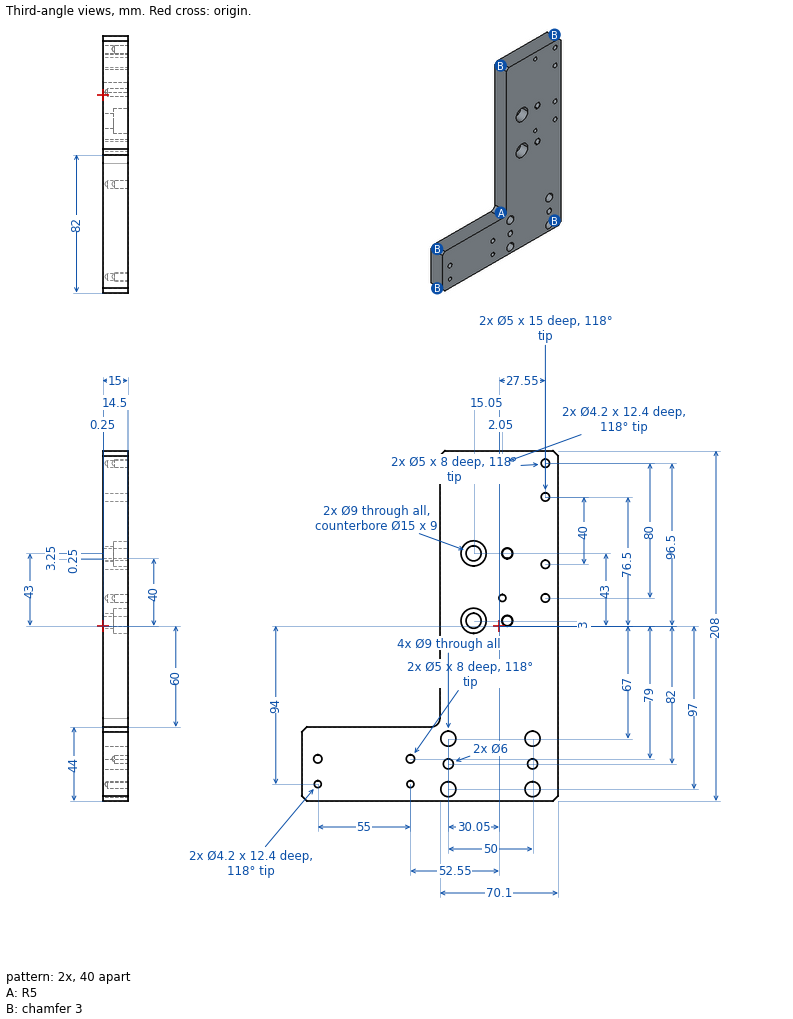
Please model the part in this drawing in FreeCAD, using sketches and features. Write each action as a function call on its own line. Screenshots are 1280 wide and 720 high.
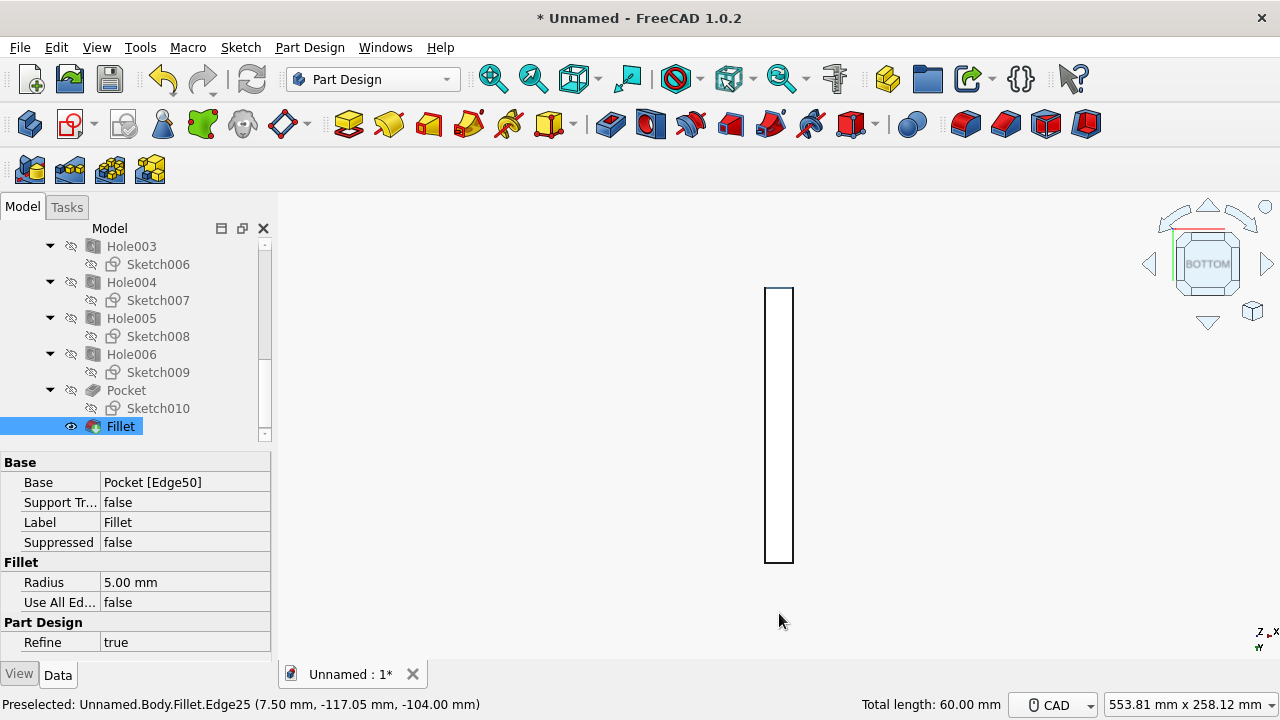
click(779, 562, ctrl)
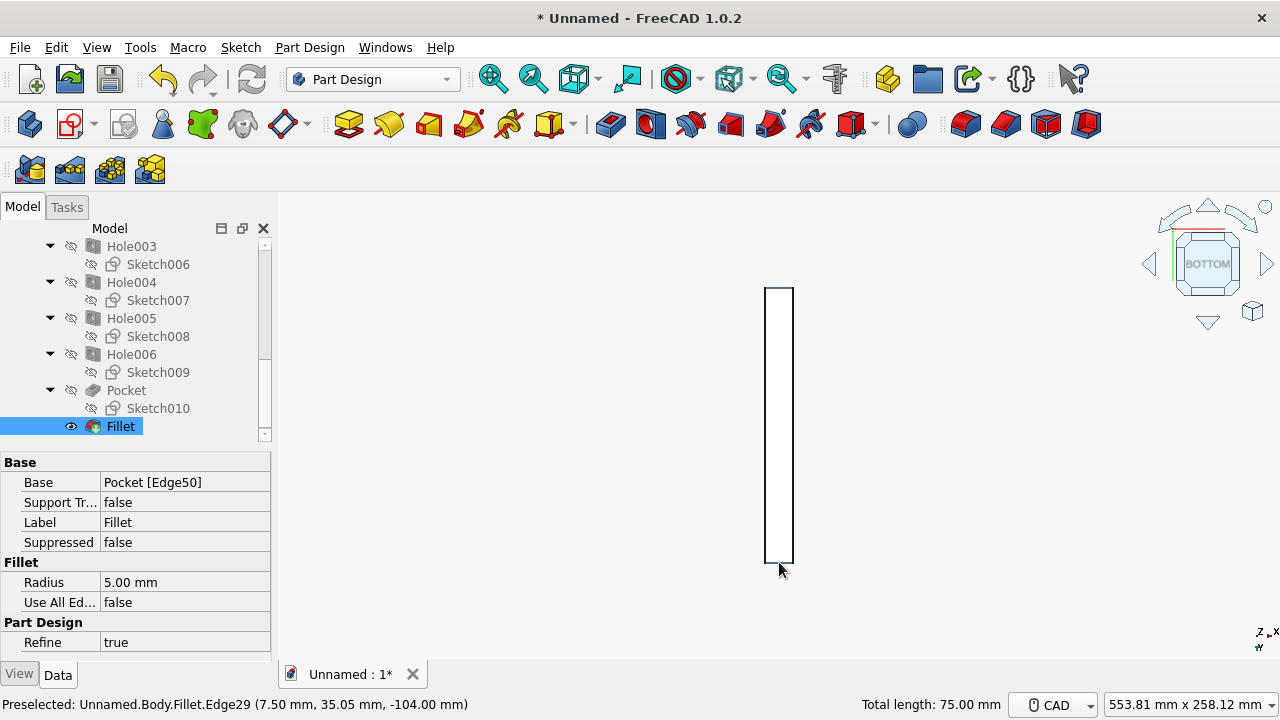
click(1006, 124)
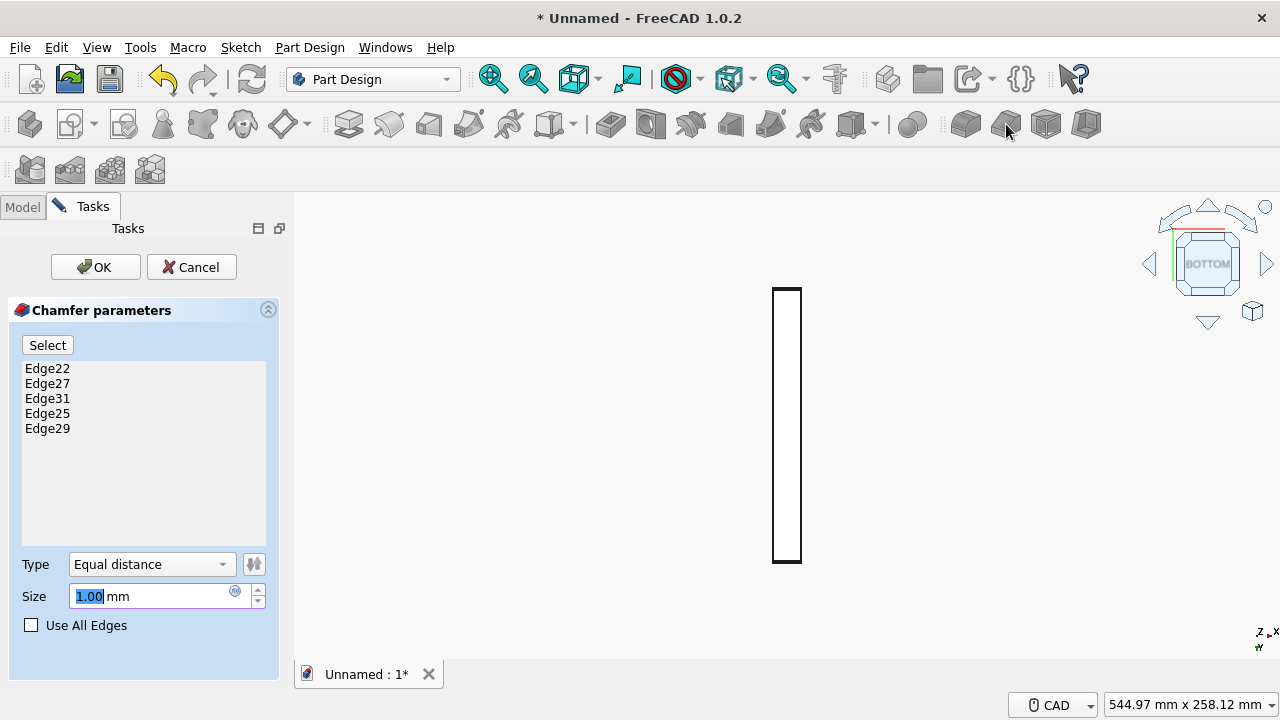
text(3)
key(Tab)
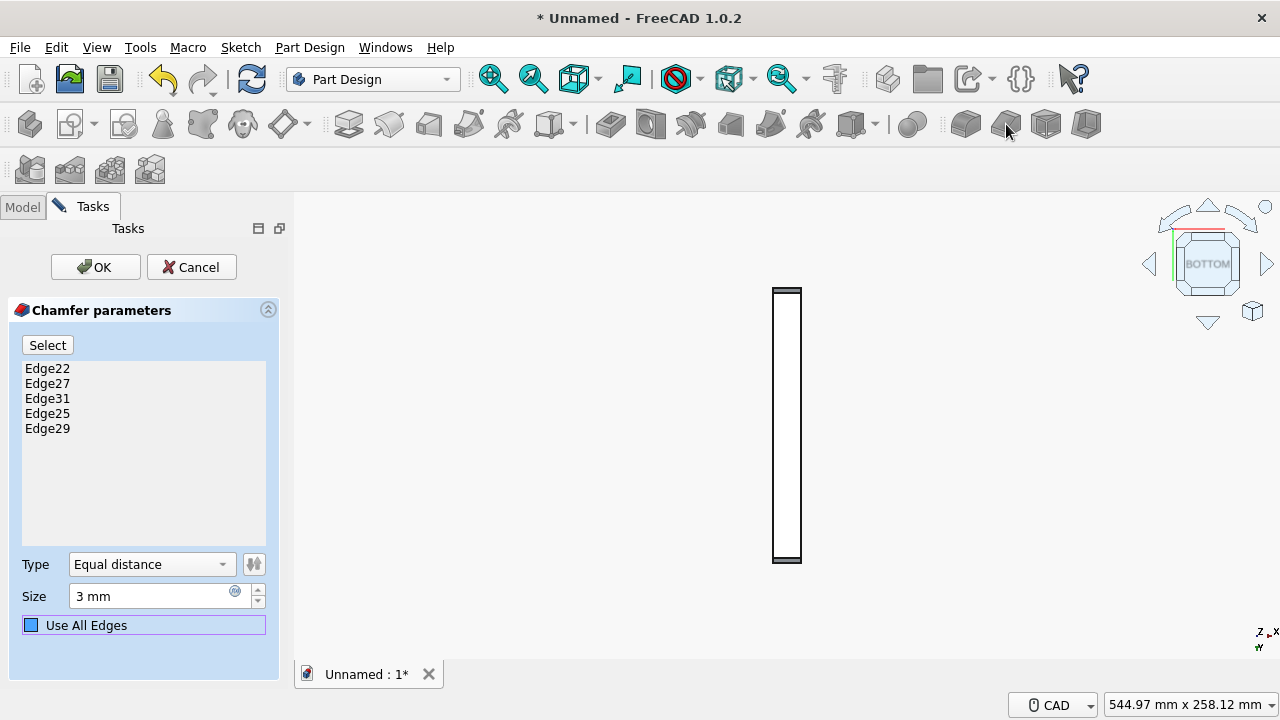
click(96, 267)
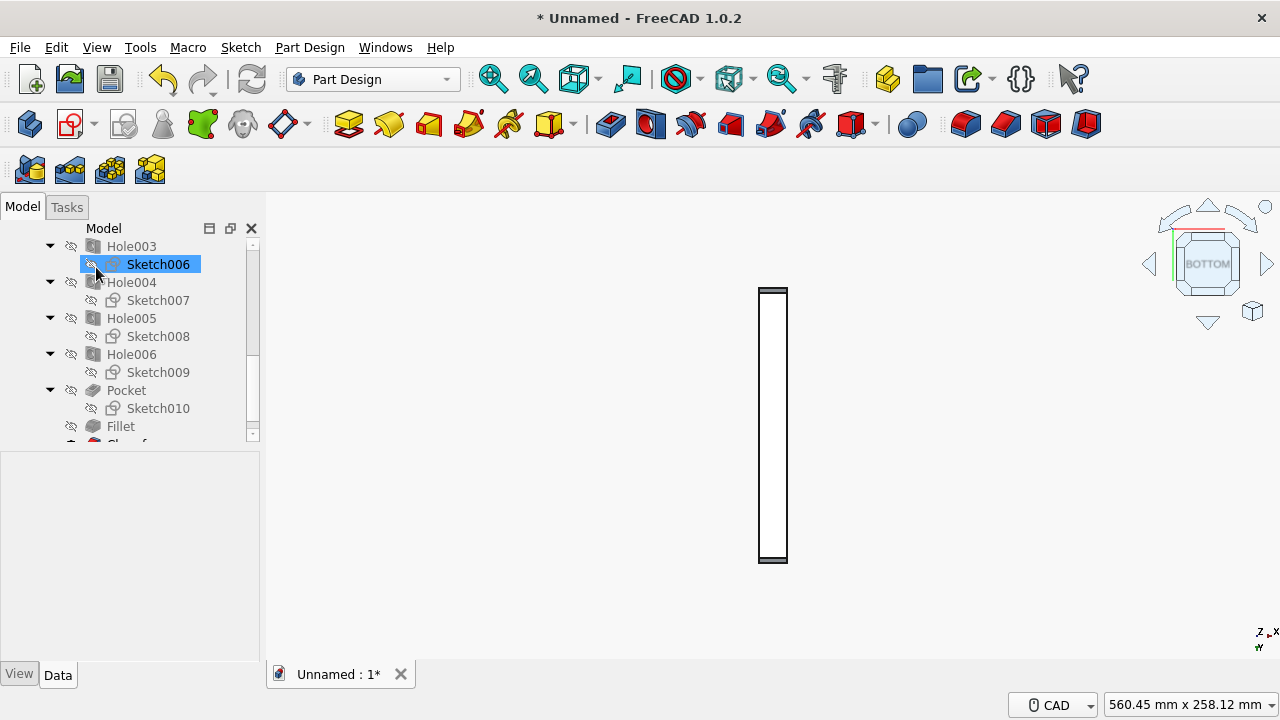
key(0)